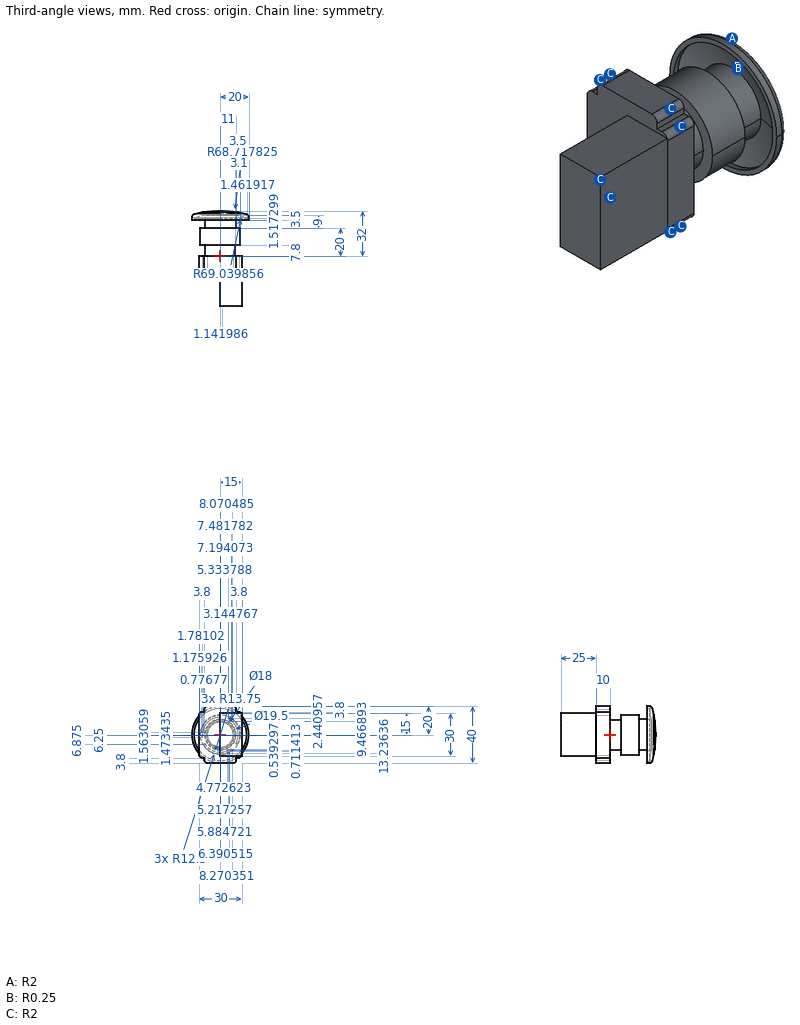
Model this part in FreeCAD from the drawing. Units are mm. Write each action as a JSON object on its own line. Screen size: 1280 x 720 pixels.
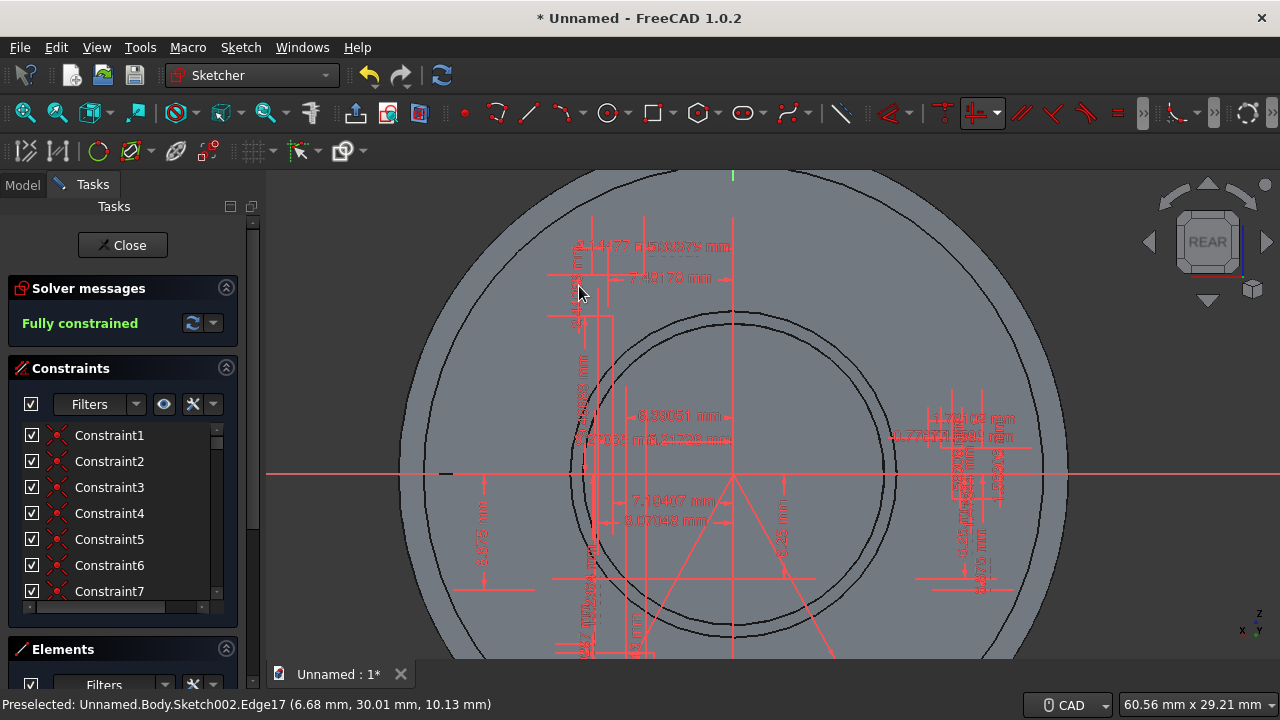
{"action": "left_click", "coordinate": [123, 245]}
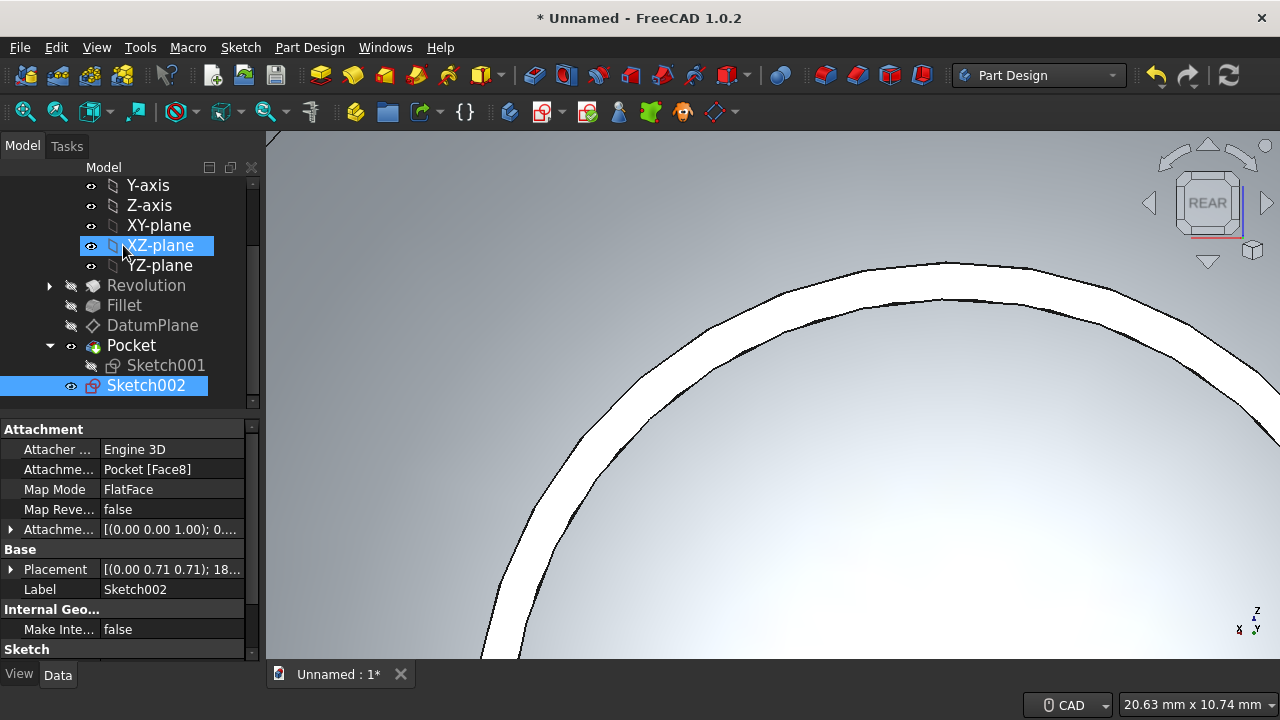
{"action": "left_click", "coordinate": [536, 76]}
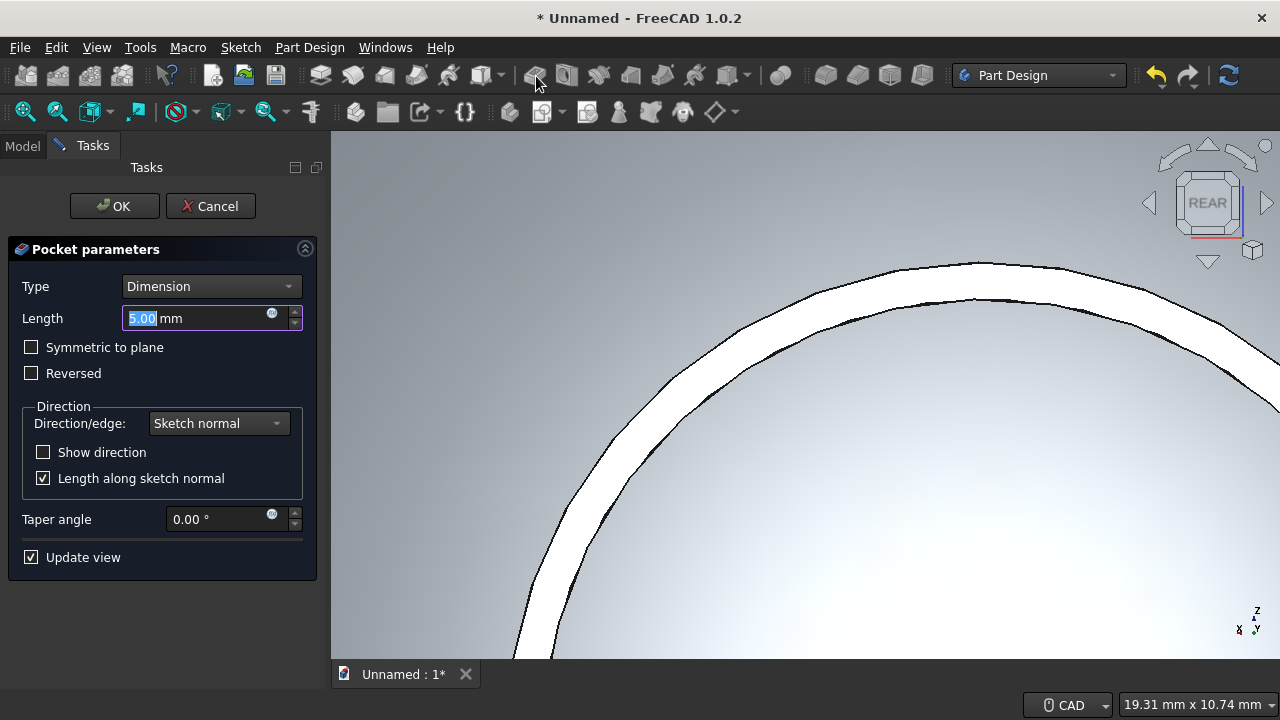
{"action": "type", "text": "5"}
{"action": "key", "text": "Tab"}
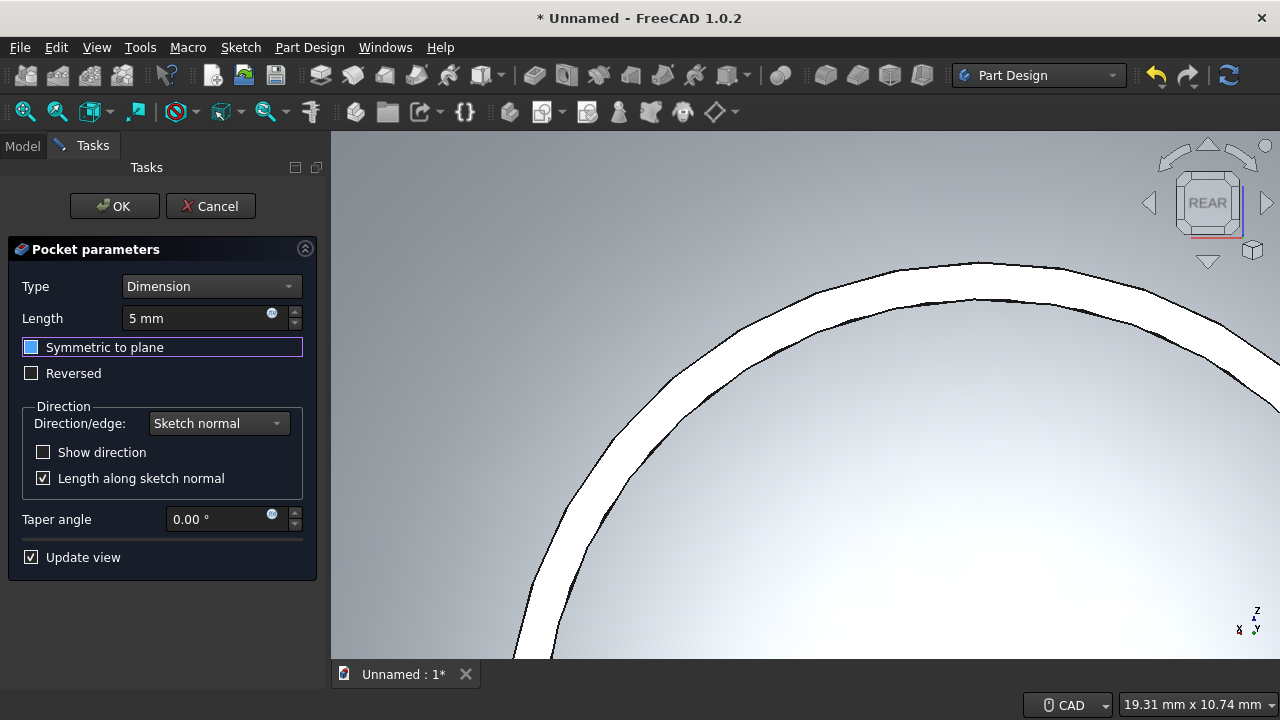
{"action": "left_click", "coordinate": [30, 373]}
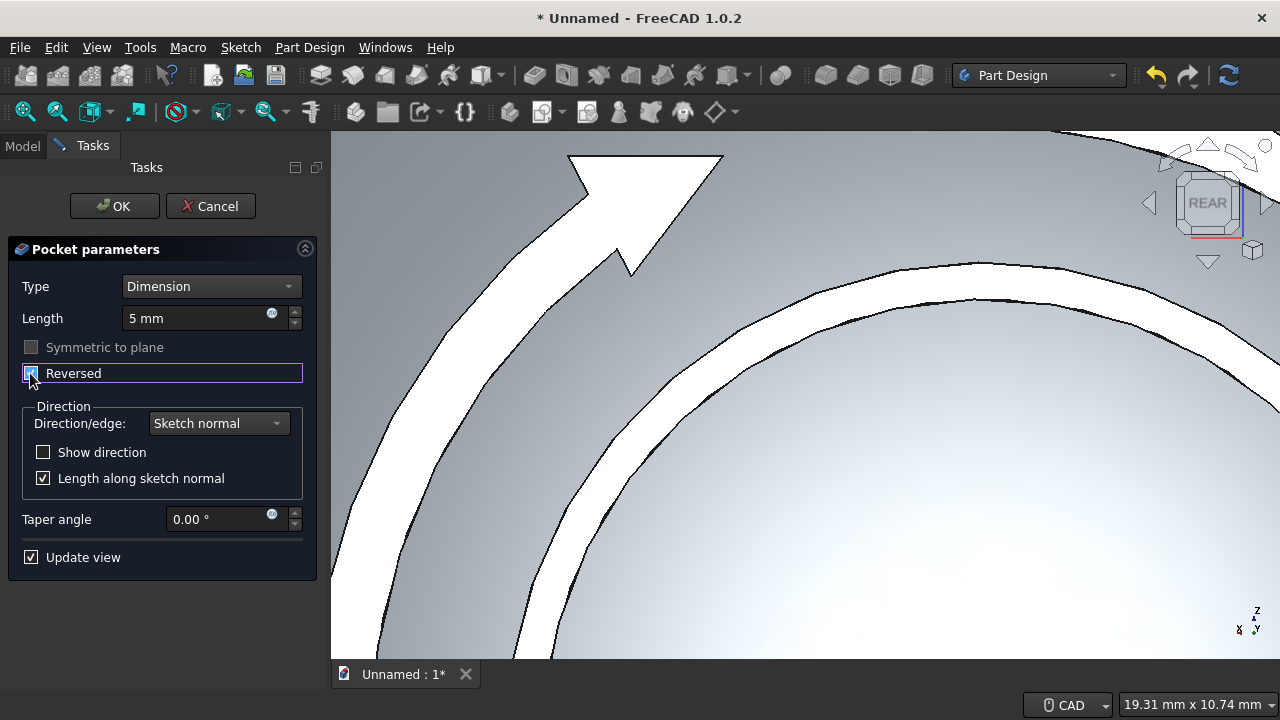
{"action": "left_click", "coordinate": [115, 206]}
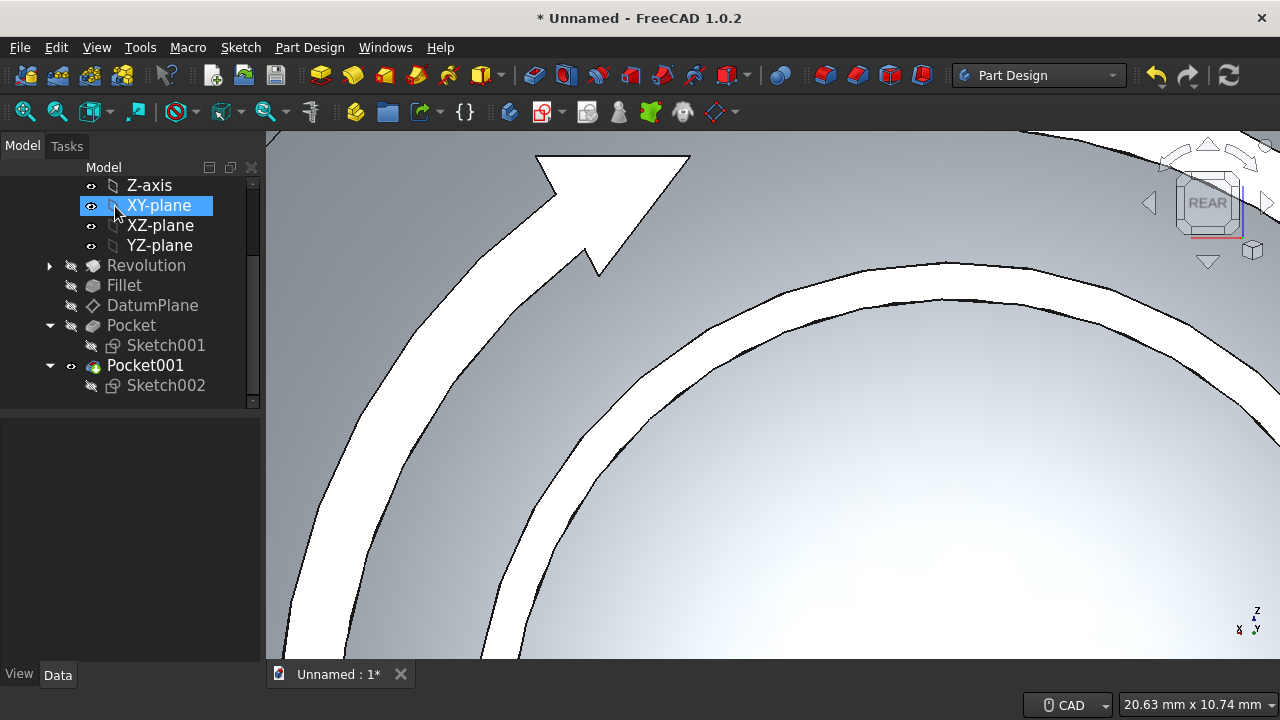
{"action": "left_click", "coordinate": [26, 112]}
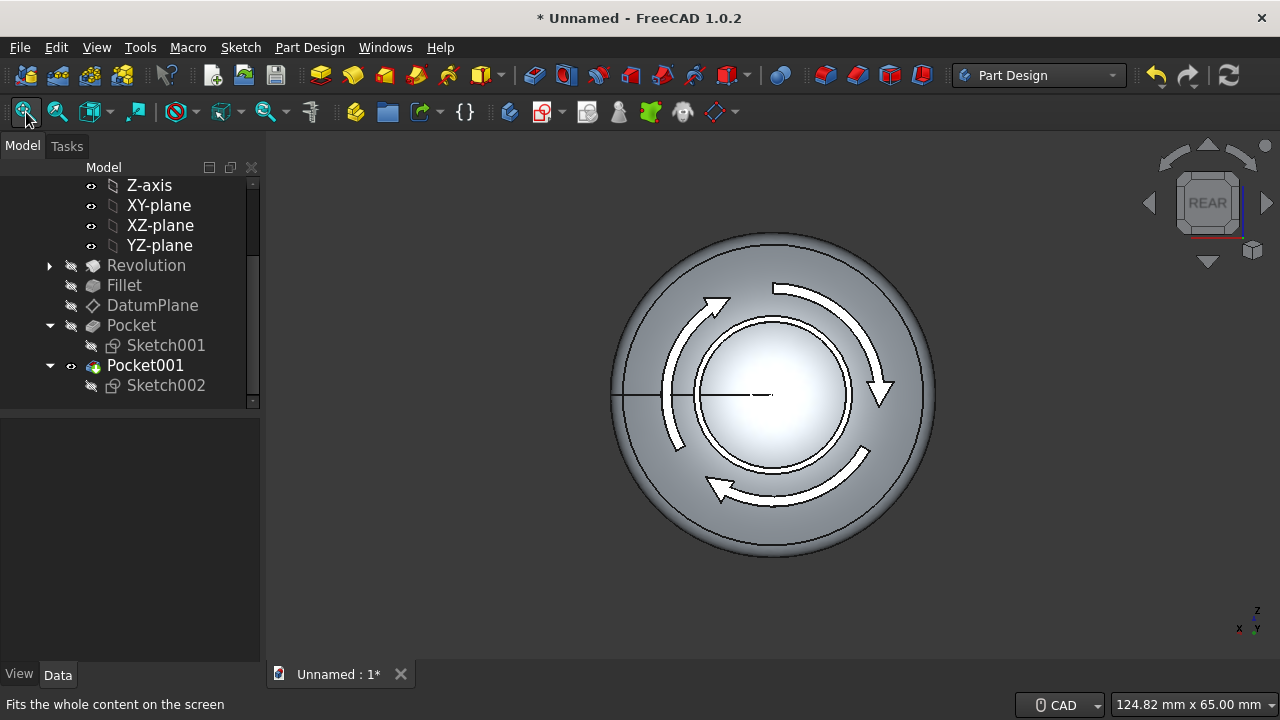
{"action": "left_click", "coordinate": [852, 394]}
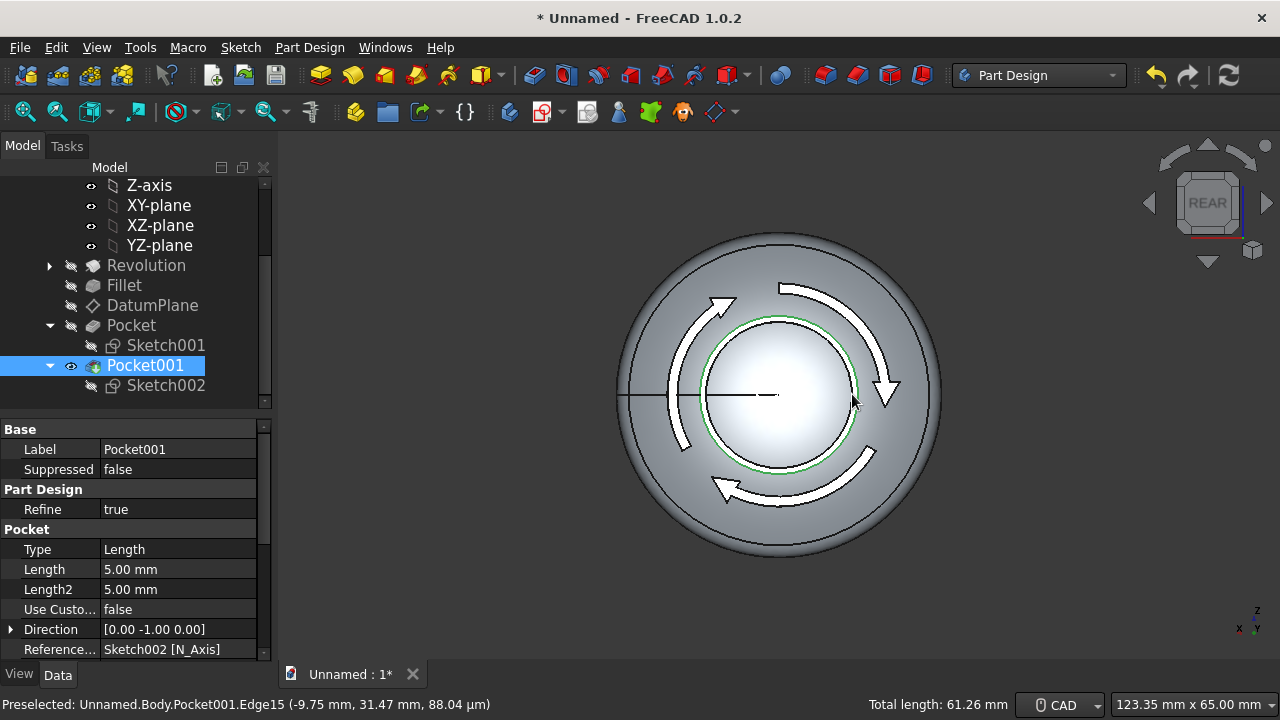
{"action": "key", "text": "0"}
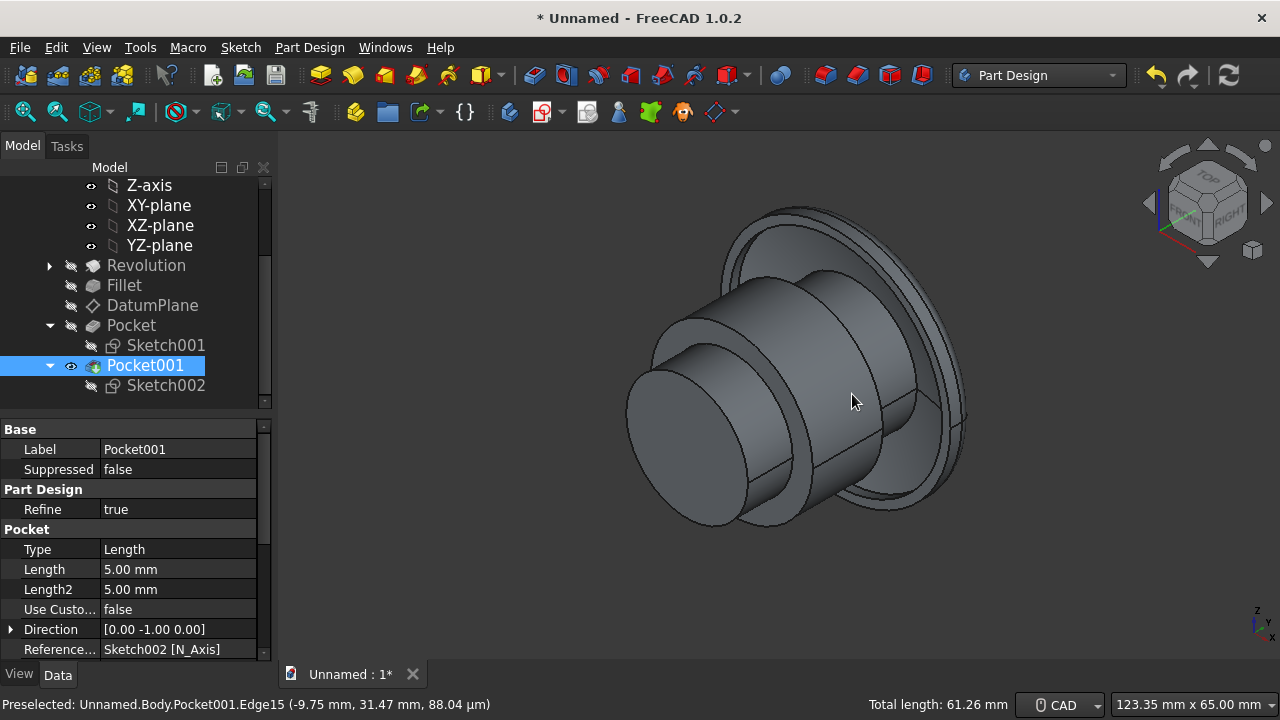
{"action": "key", "text": "2"}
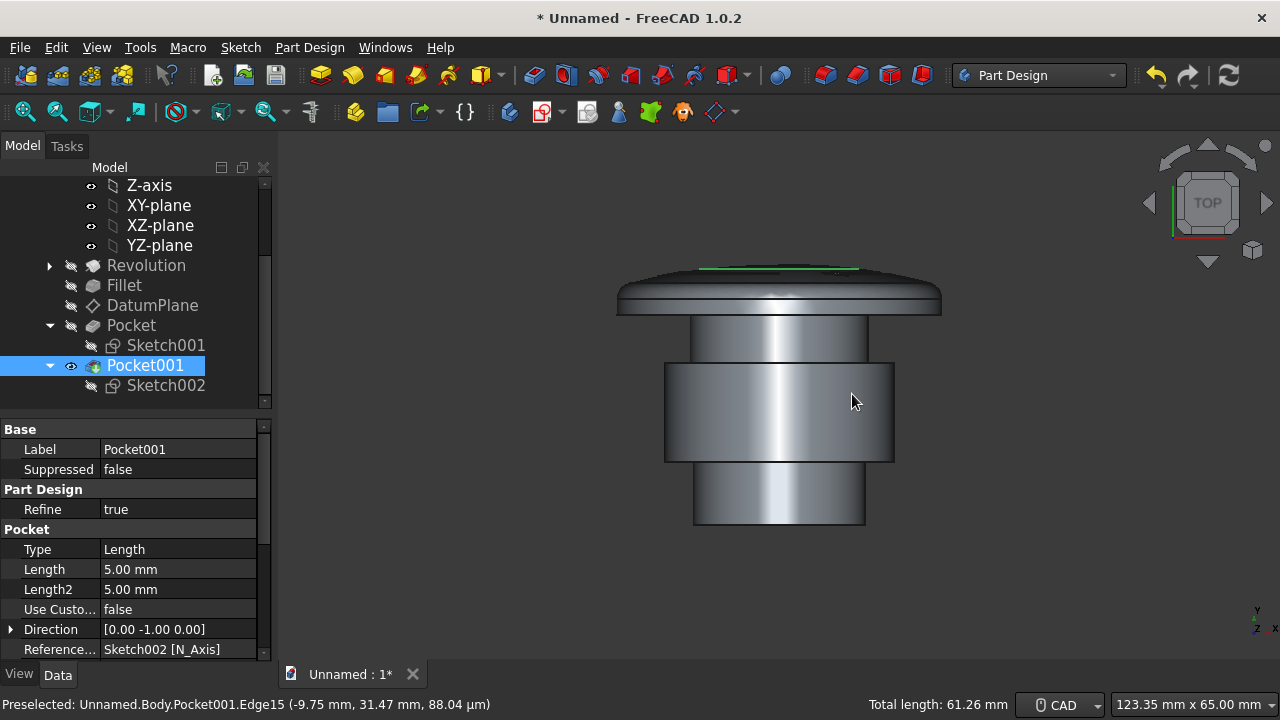
{"action": "key", "text": "1"}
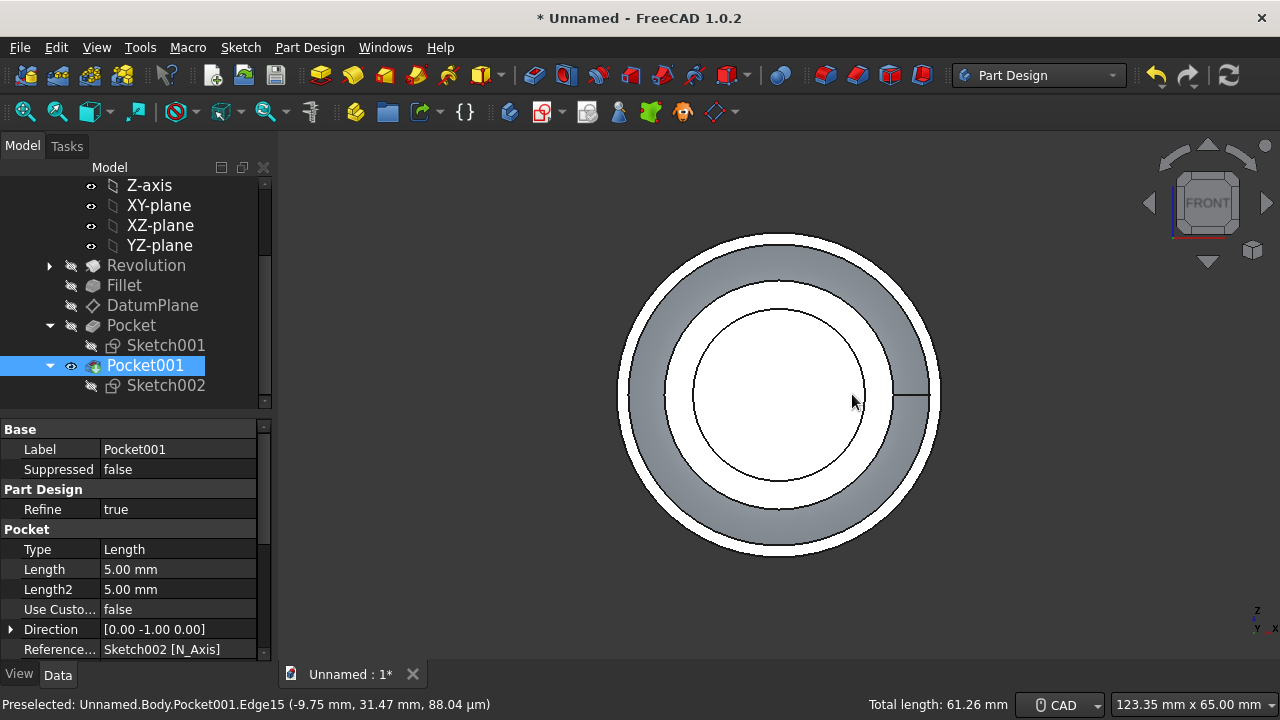
{"action": "key", "text": "3"}